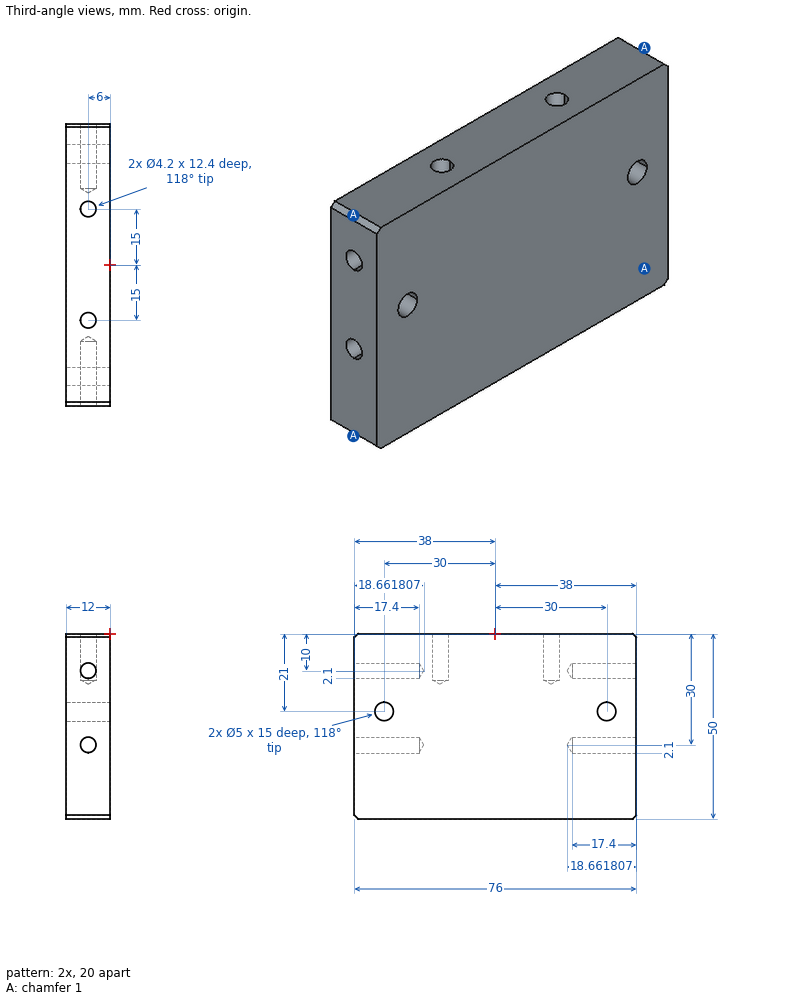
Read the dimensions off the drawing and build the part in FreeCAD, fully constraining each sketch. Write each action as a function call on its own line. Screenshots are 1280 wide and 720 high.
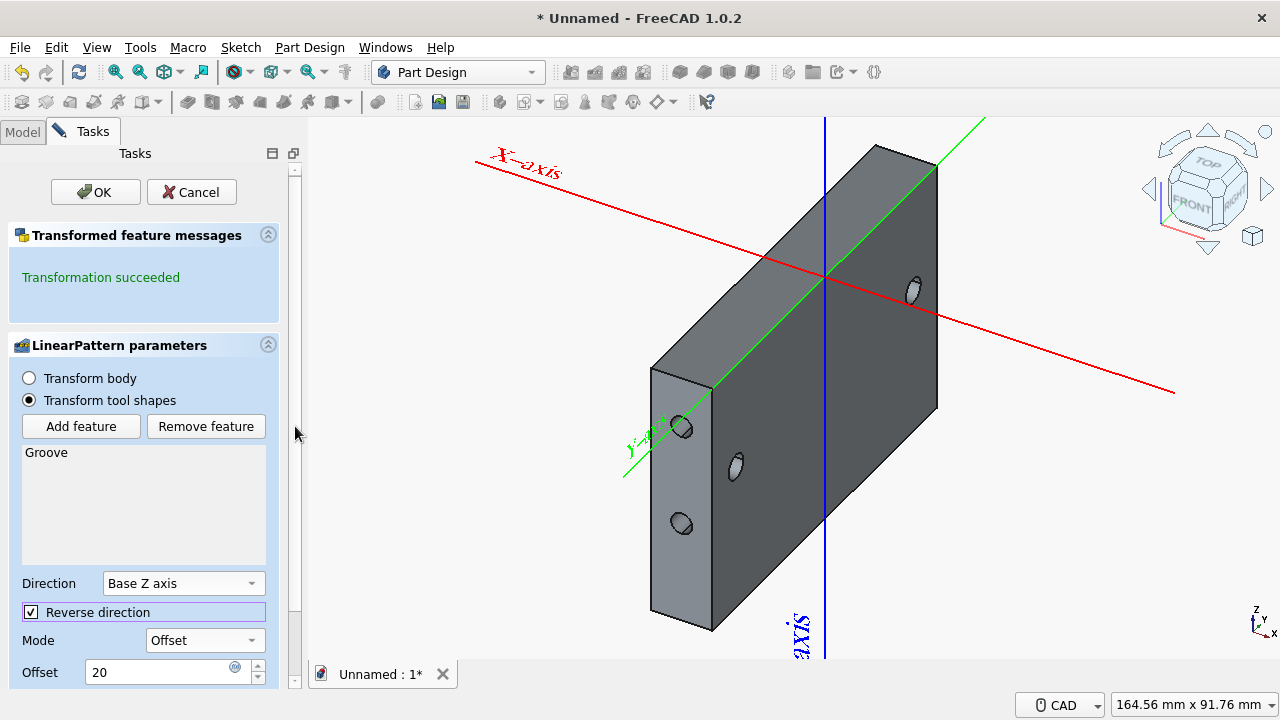
click(96, 192)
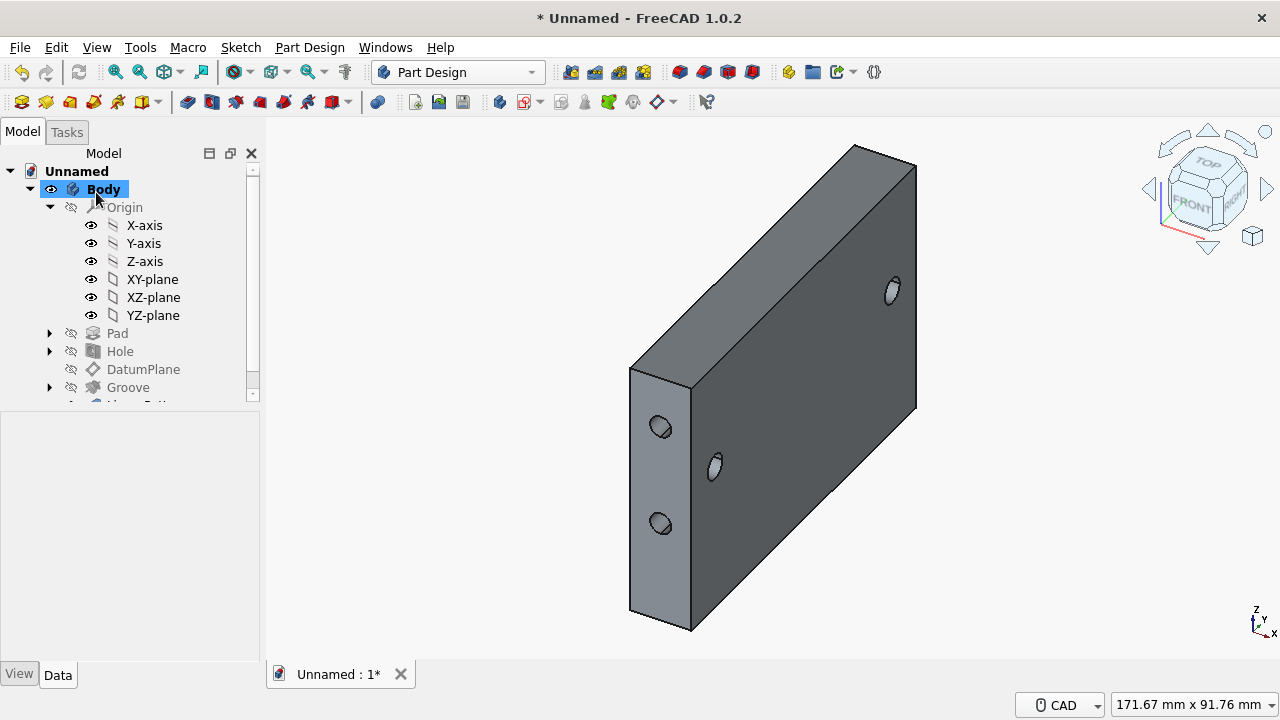
click(116, 387)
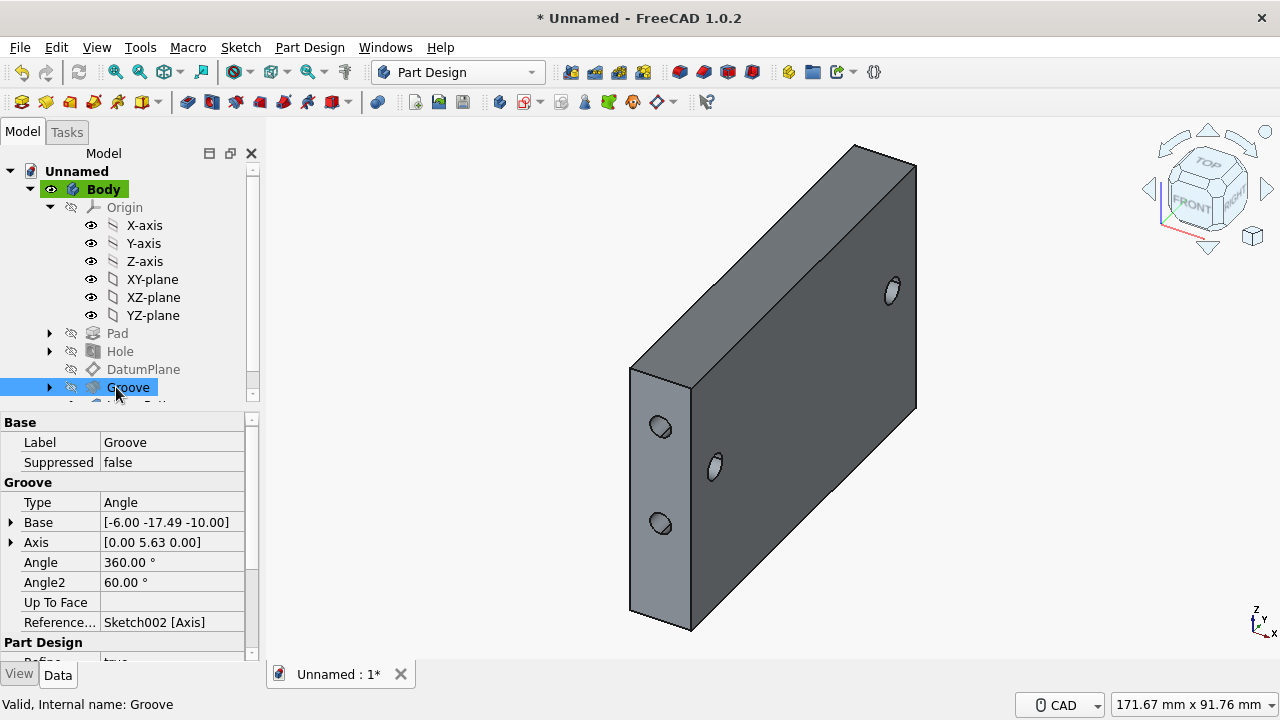
click(572, 72)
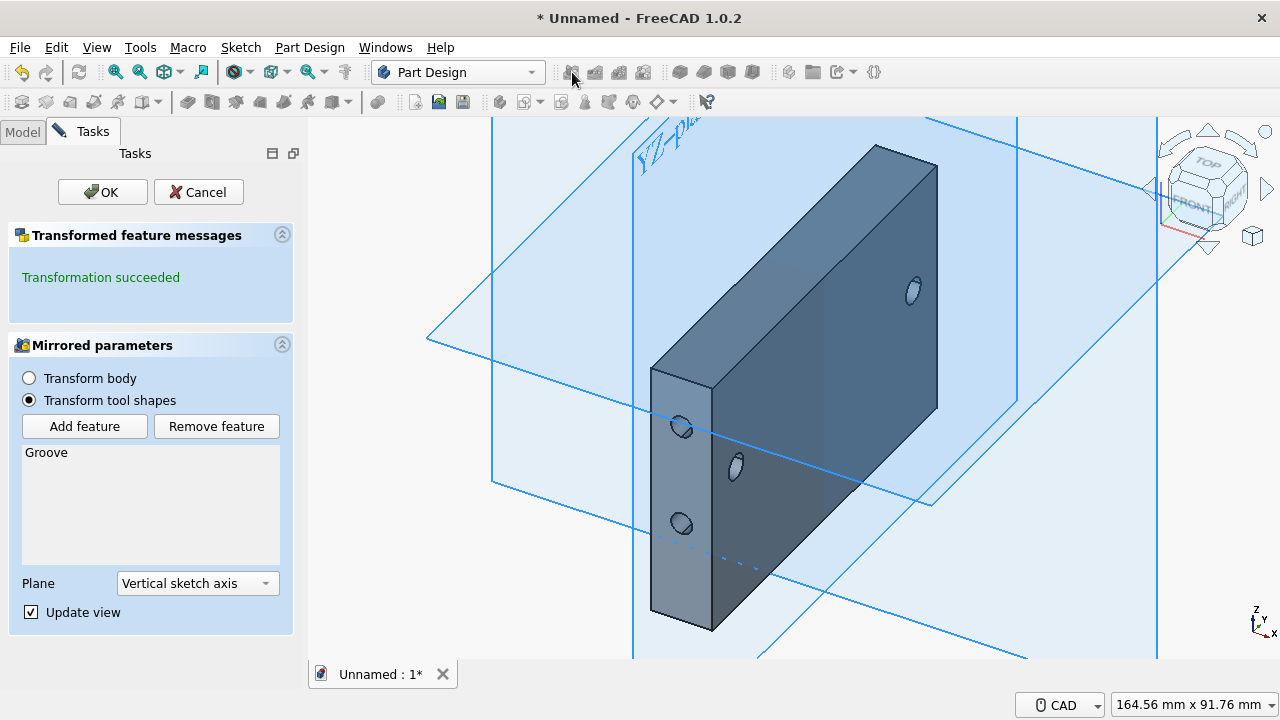
click(198, 584)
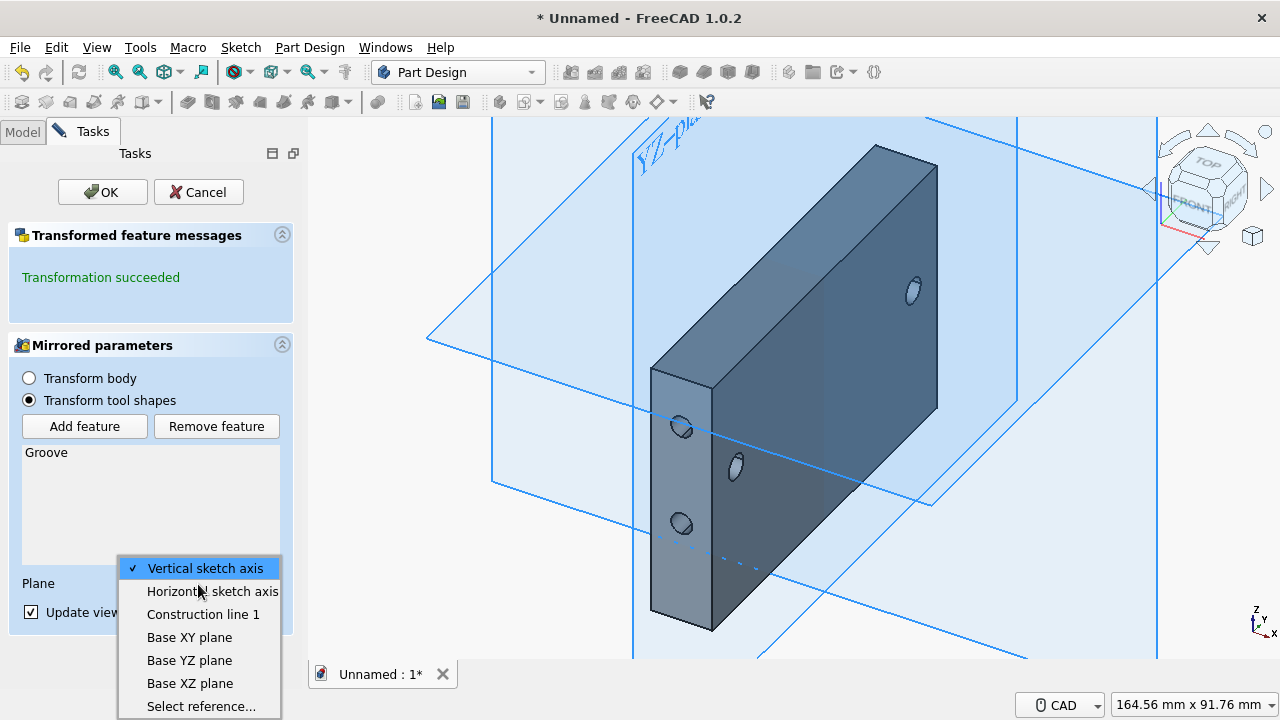
click(198, 684)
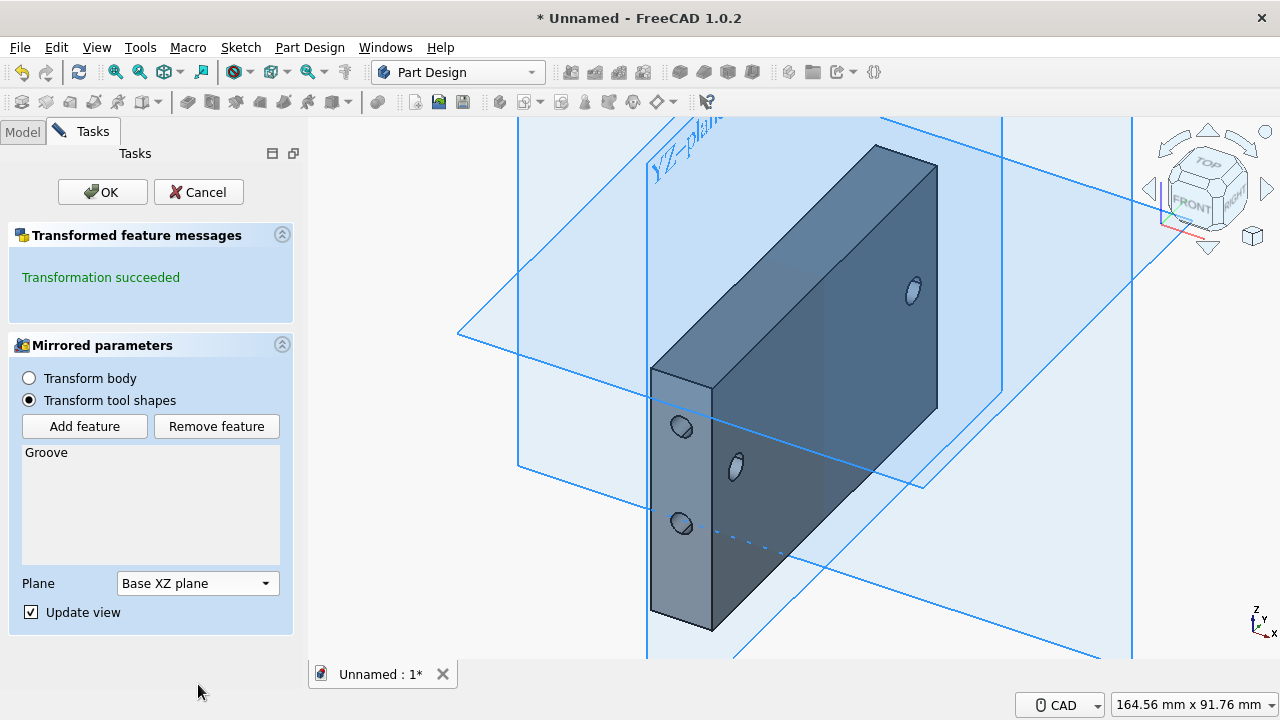
click(103, 192)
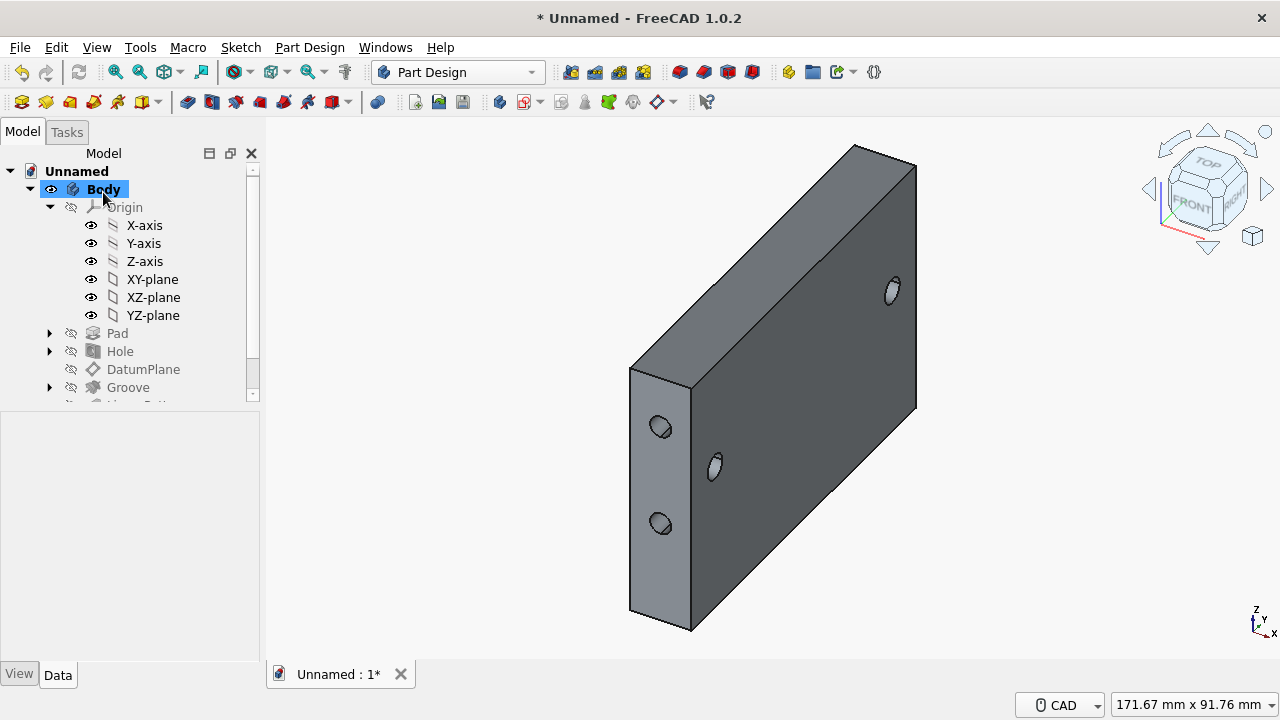
click(136, 315)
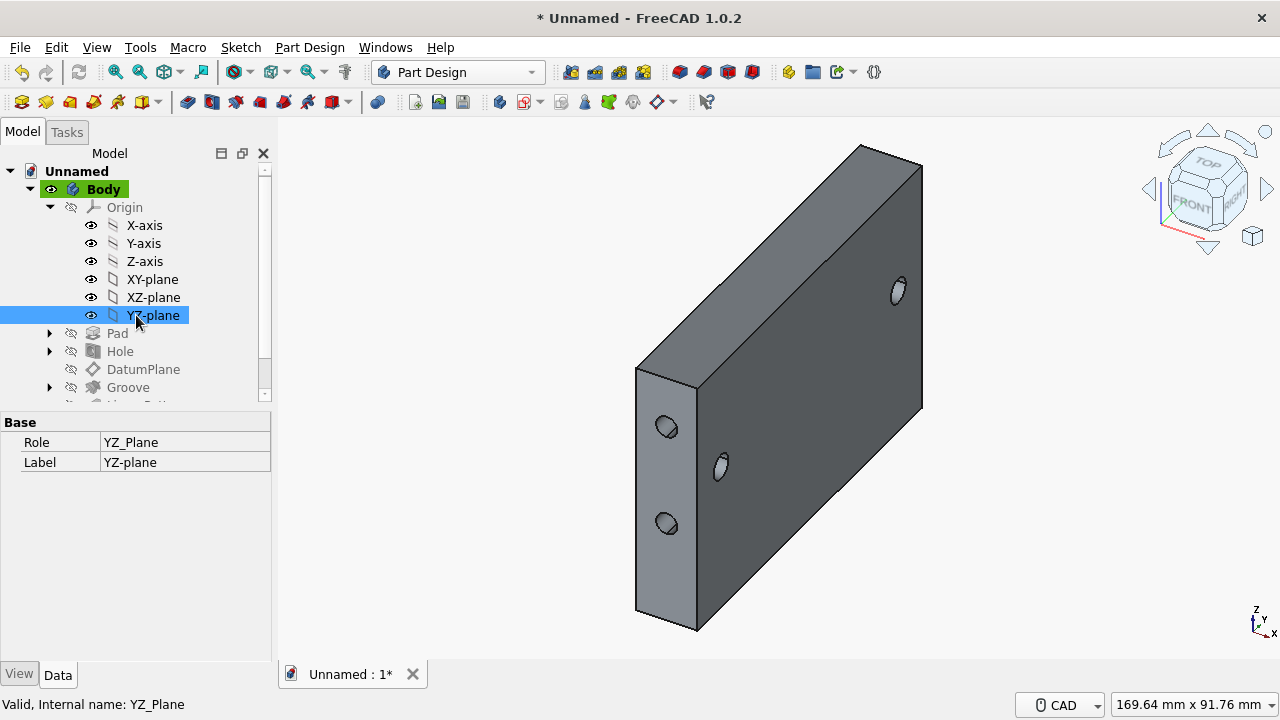
click(658, 102)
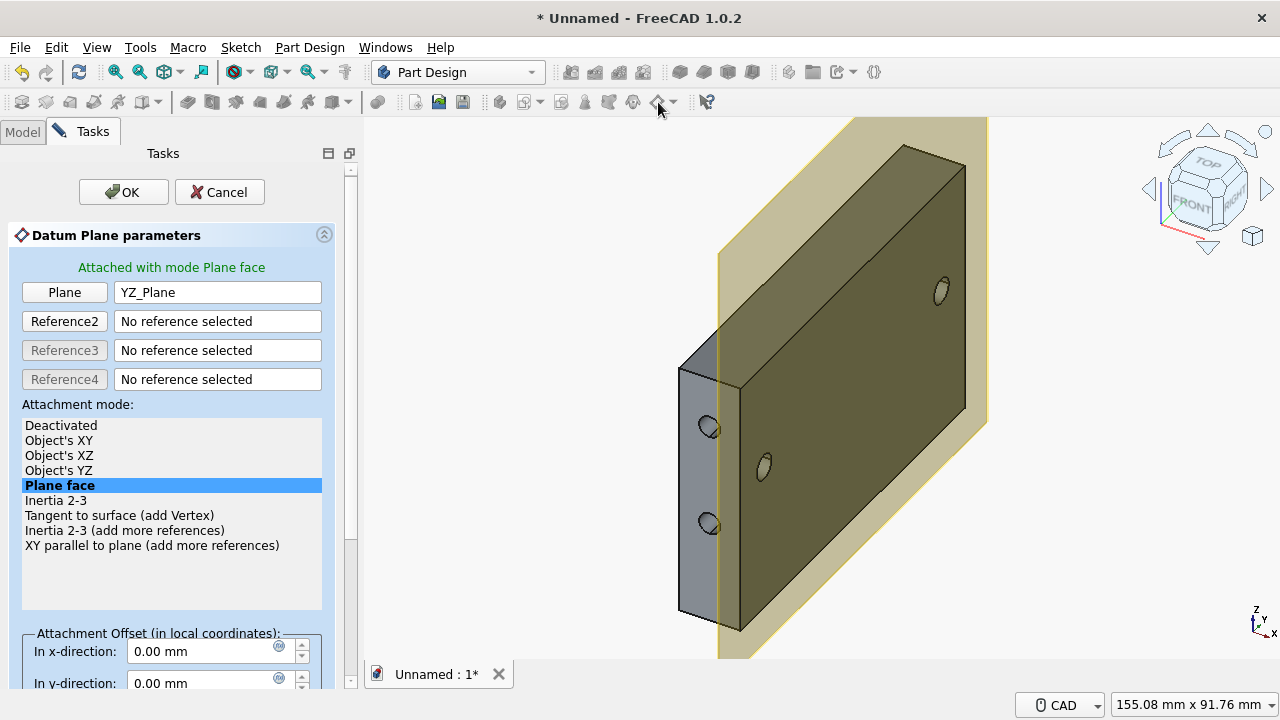
scroll(351, 426, down, 2)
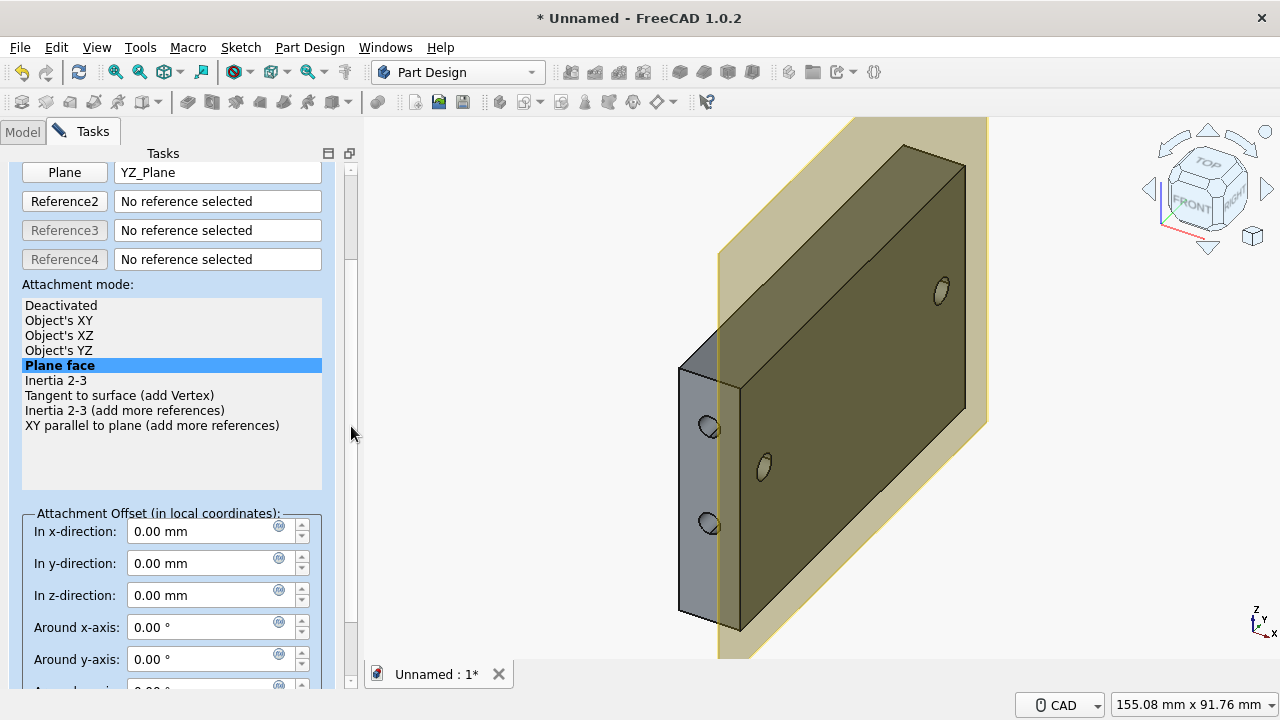
triple_click(210, 595)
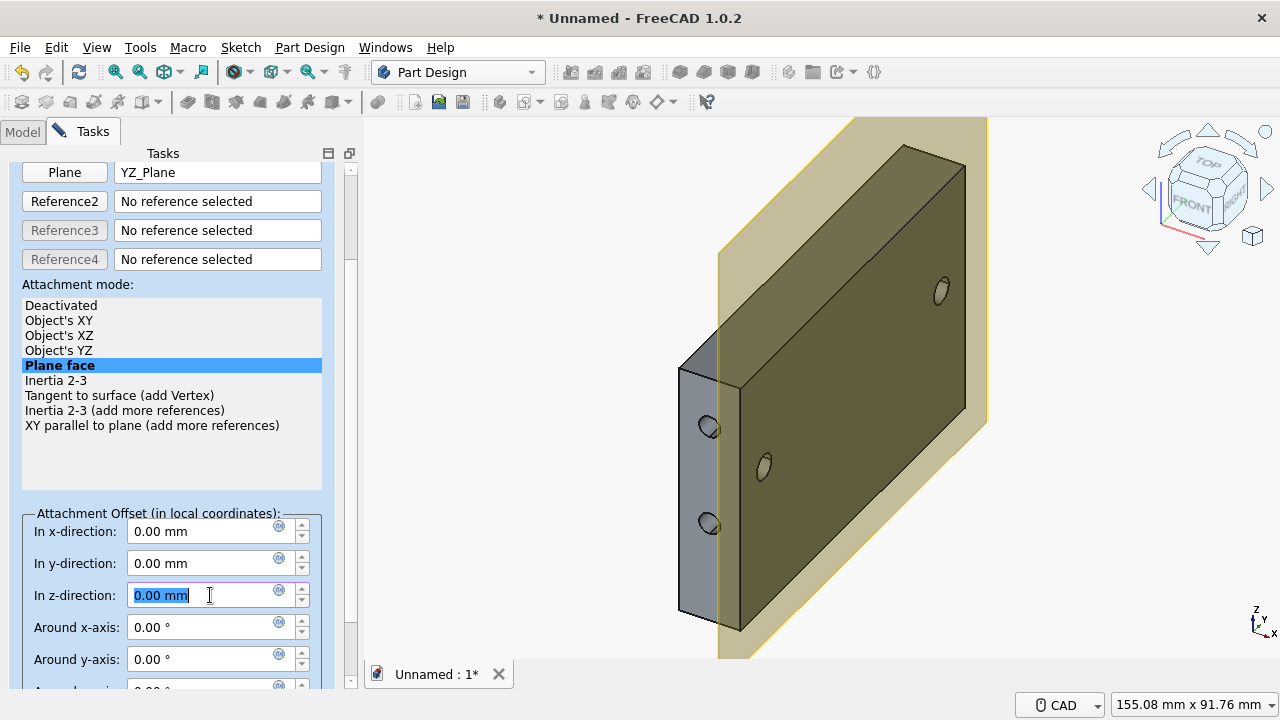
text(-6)
key(Tab)